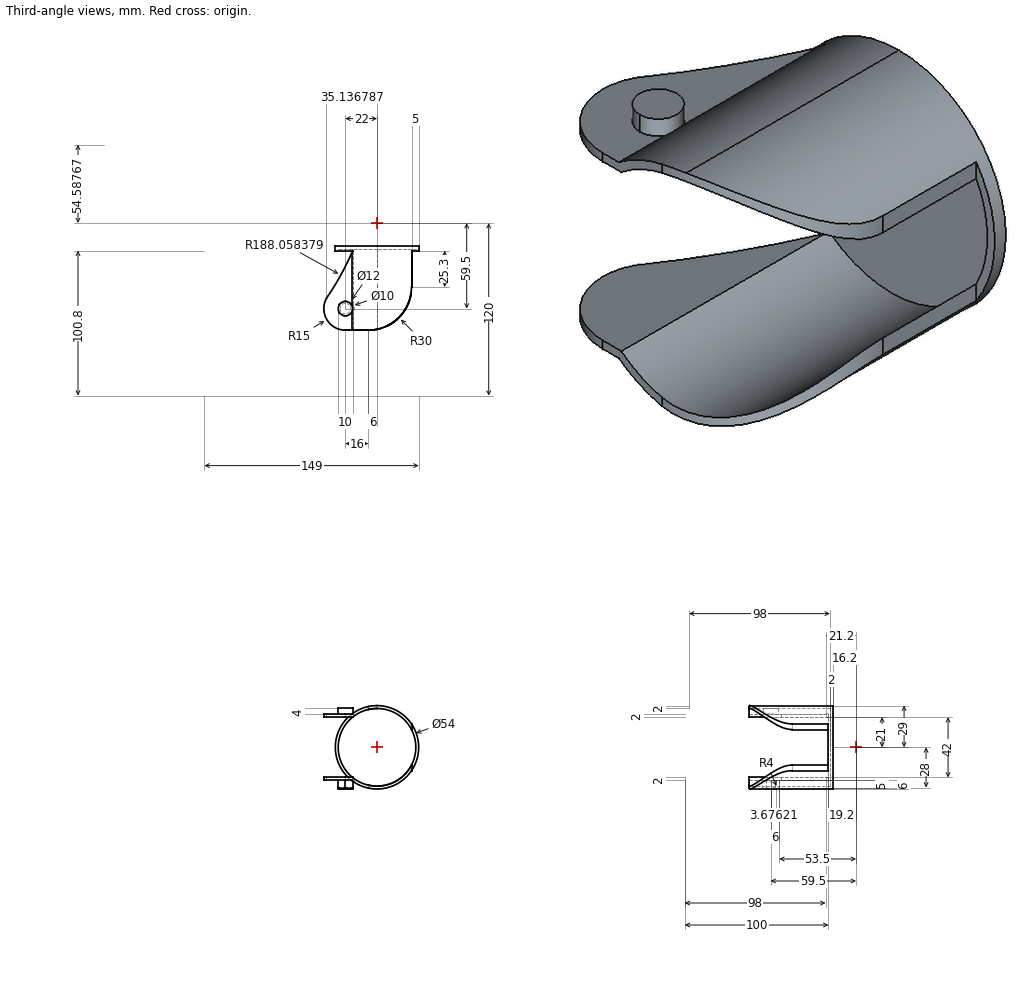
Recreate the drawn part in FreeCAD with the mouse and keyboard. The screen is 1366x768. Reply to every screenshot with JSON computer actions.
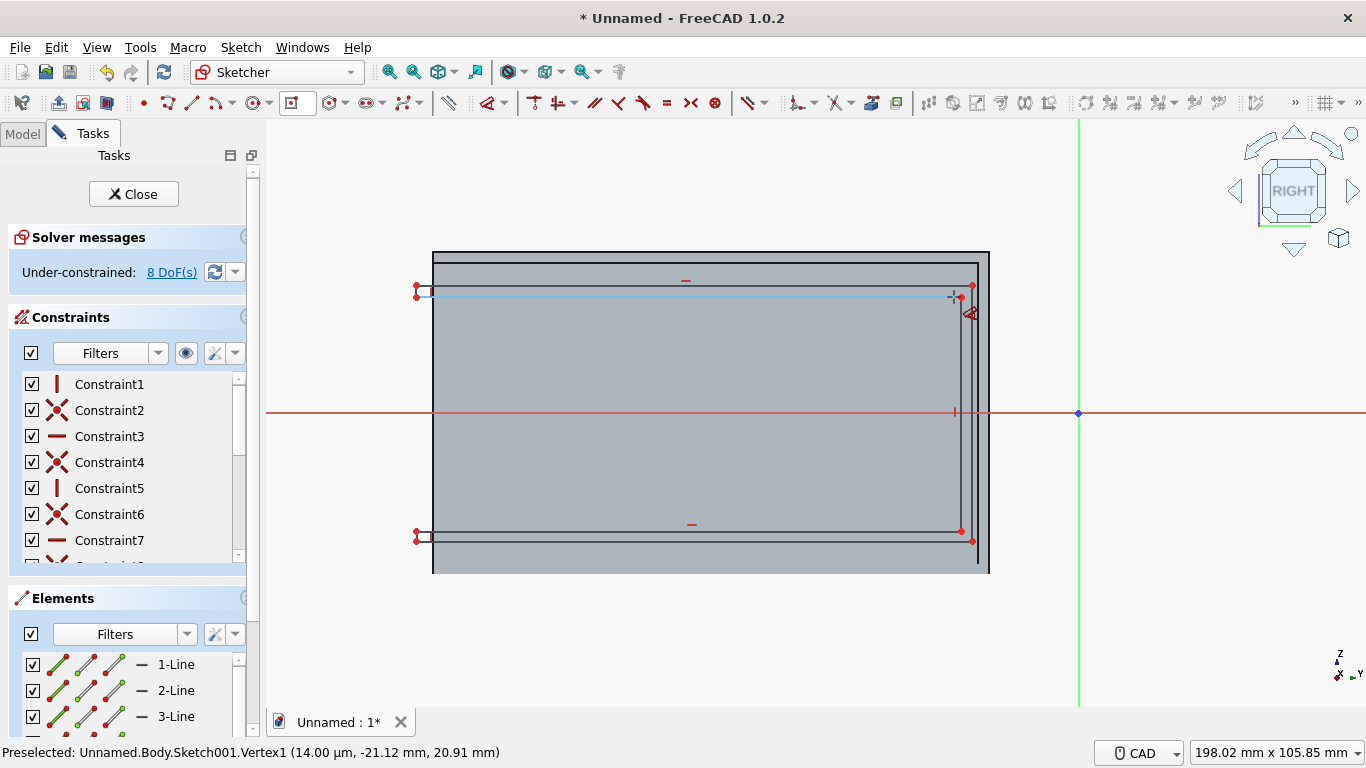
{"action": "scroll", "coordinate": [417, 537], "scroll_direction": "up", "scroll_amount": 7}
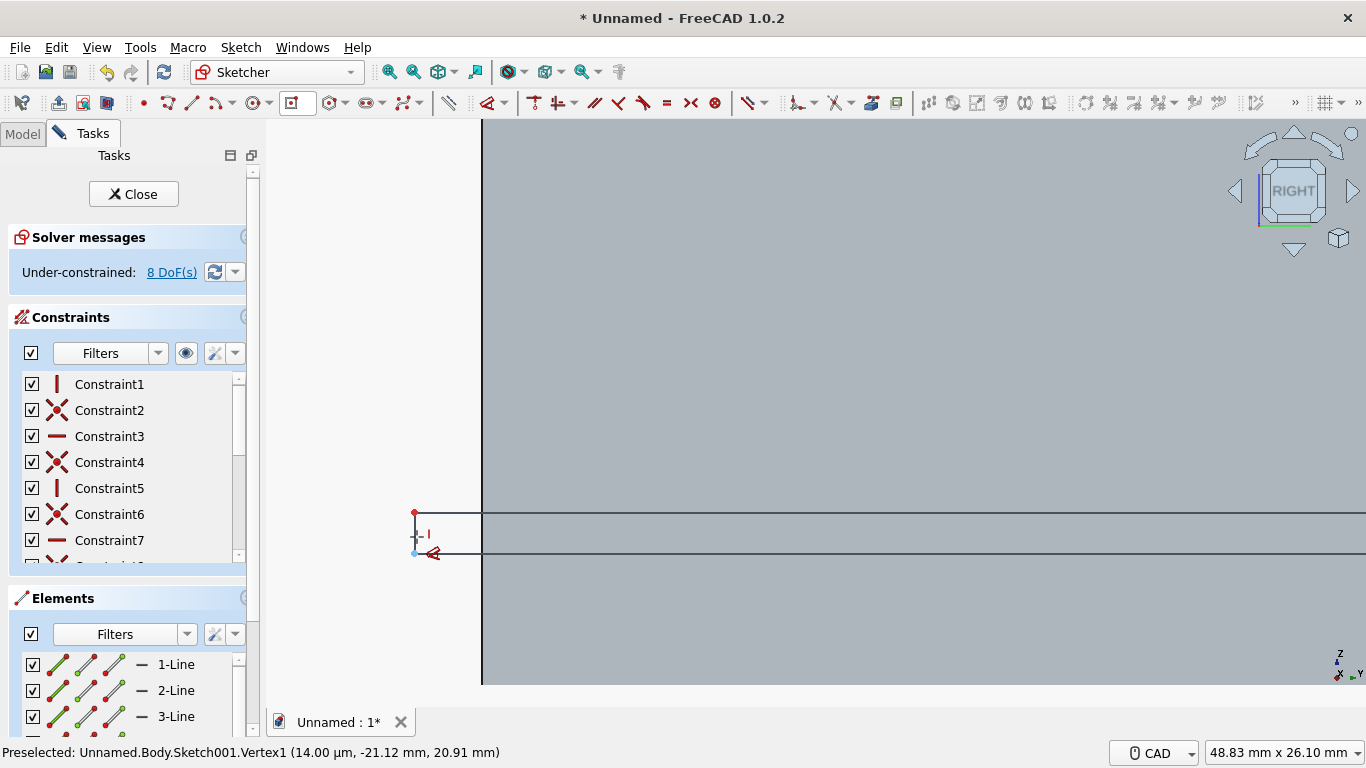
{"action": "left_click", "coordinate": [415, 533]}
{"action": "left_click", "coordinate": [381, 533]}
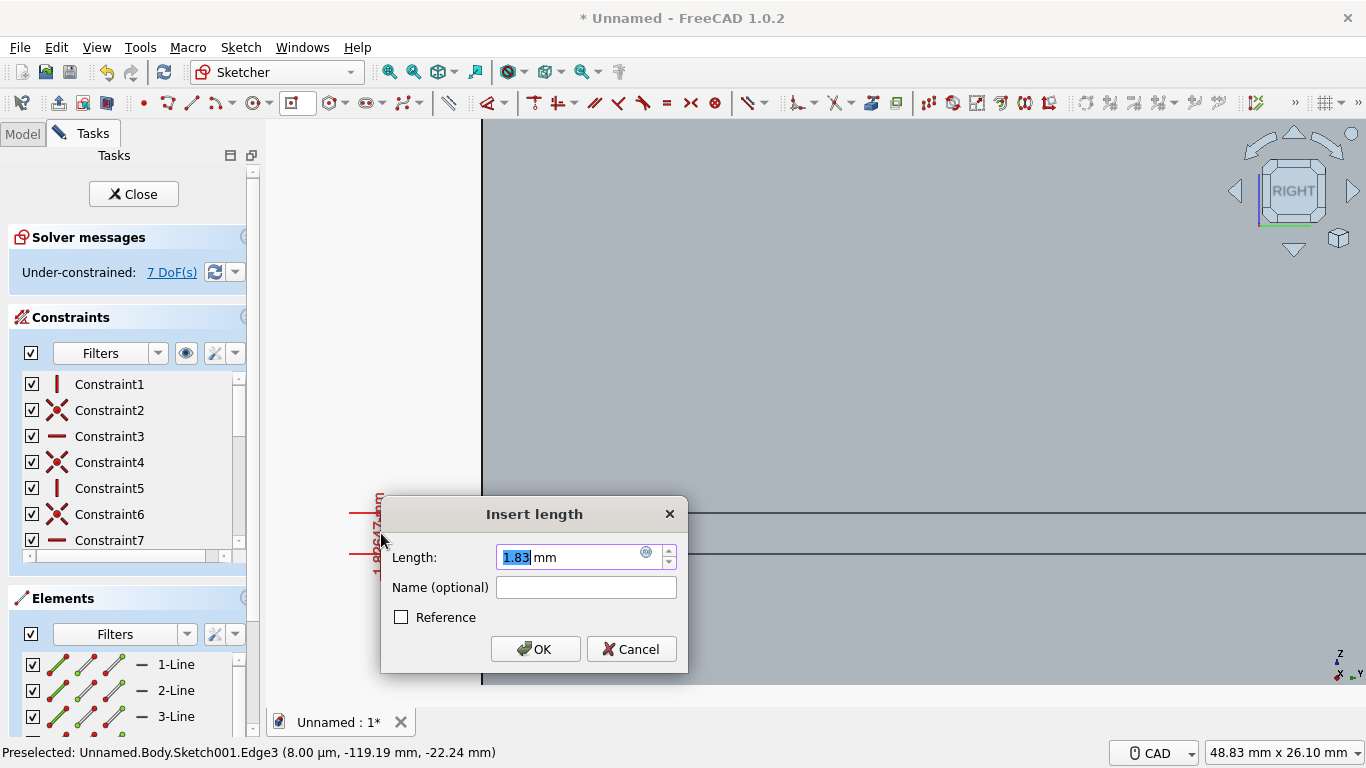
{"action": "type", "text": "2"}
{"action": "key", "text": "Return"}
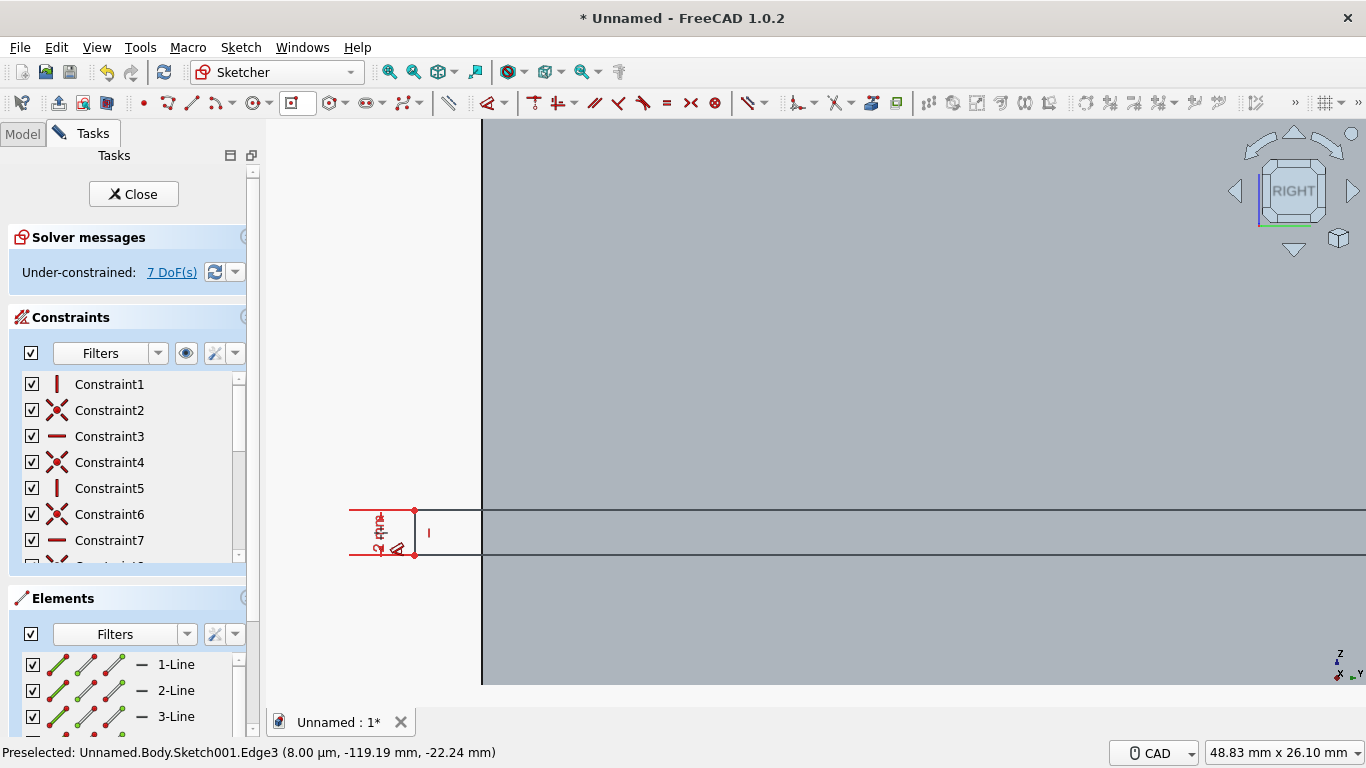
{"action": "scroll", "coordinate": [417, 537], "scroll_direction": "down", "scroll_amount": 7}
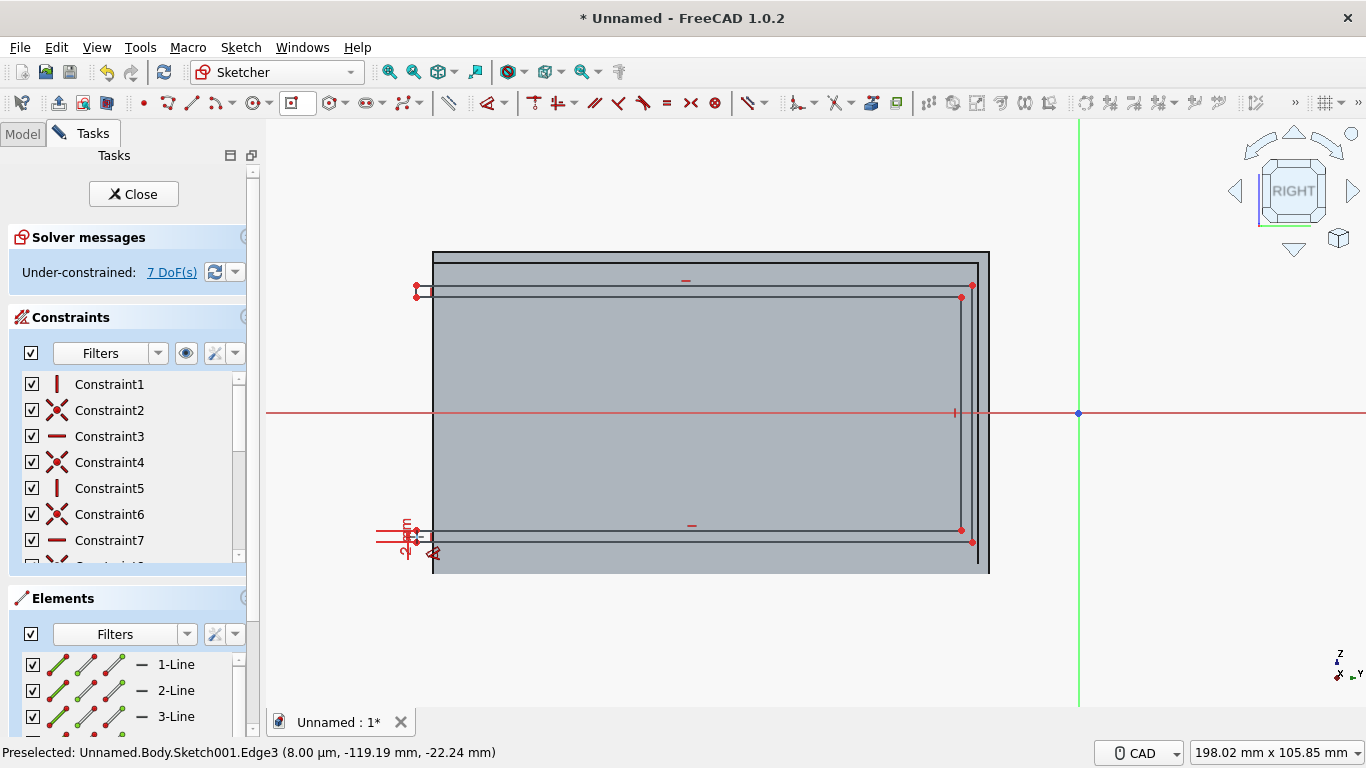
{"action": "scroll", "coordinate": [416, 289], "scroll_direction": "up", "scroll_amount": 8}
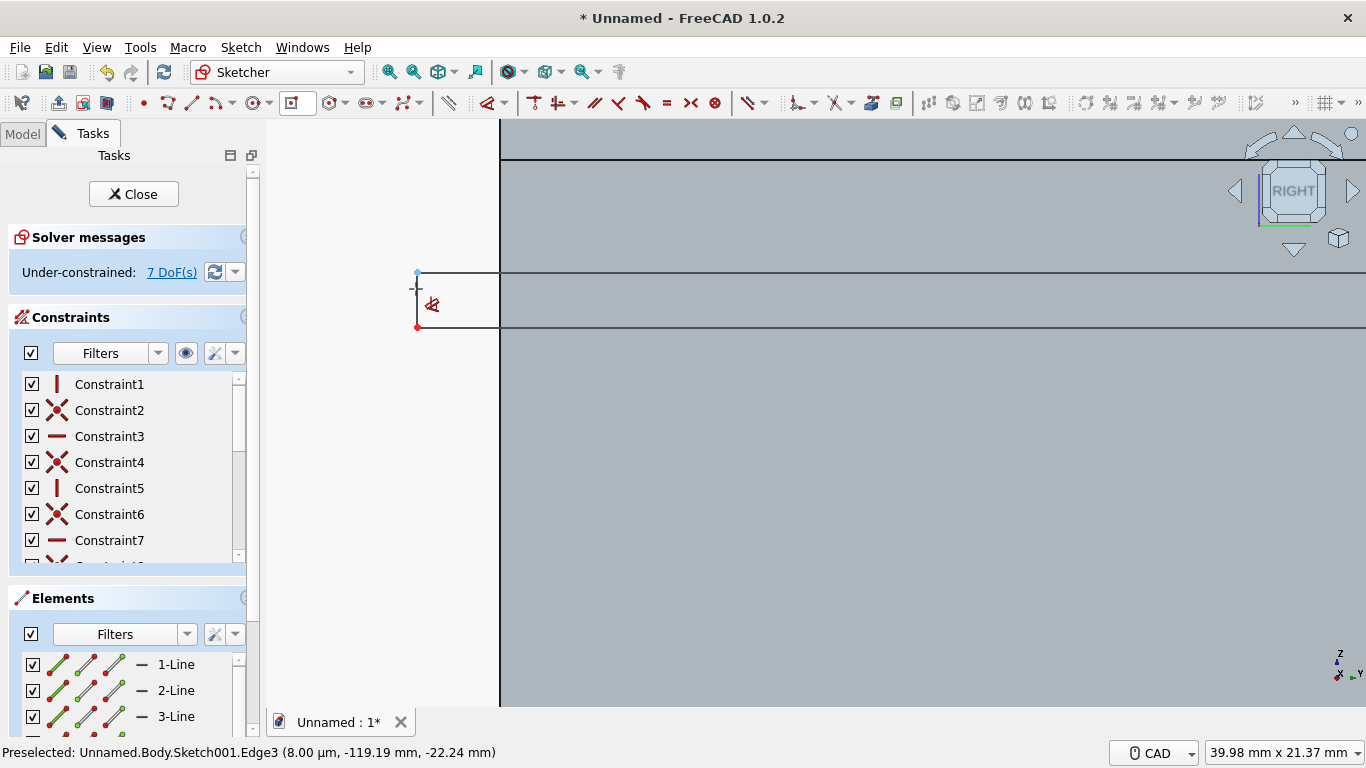
{"action": "left_click", "coordinate": [417, 289]}
{"action": "left_click", "coordinate": [383, 300]}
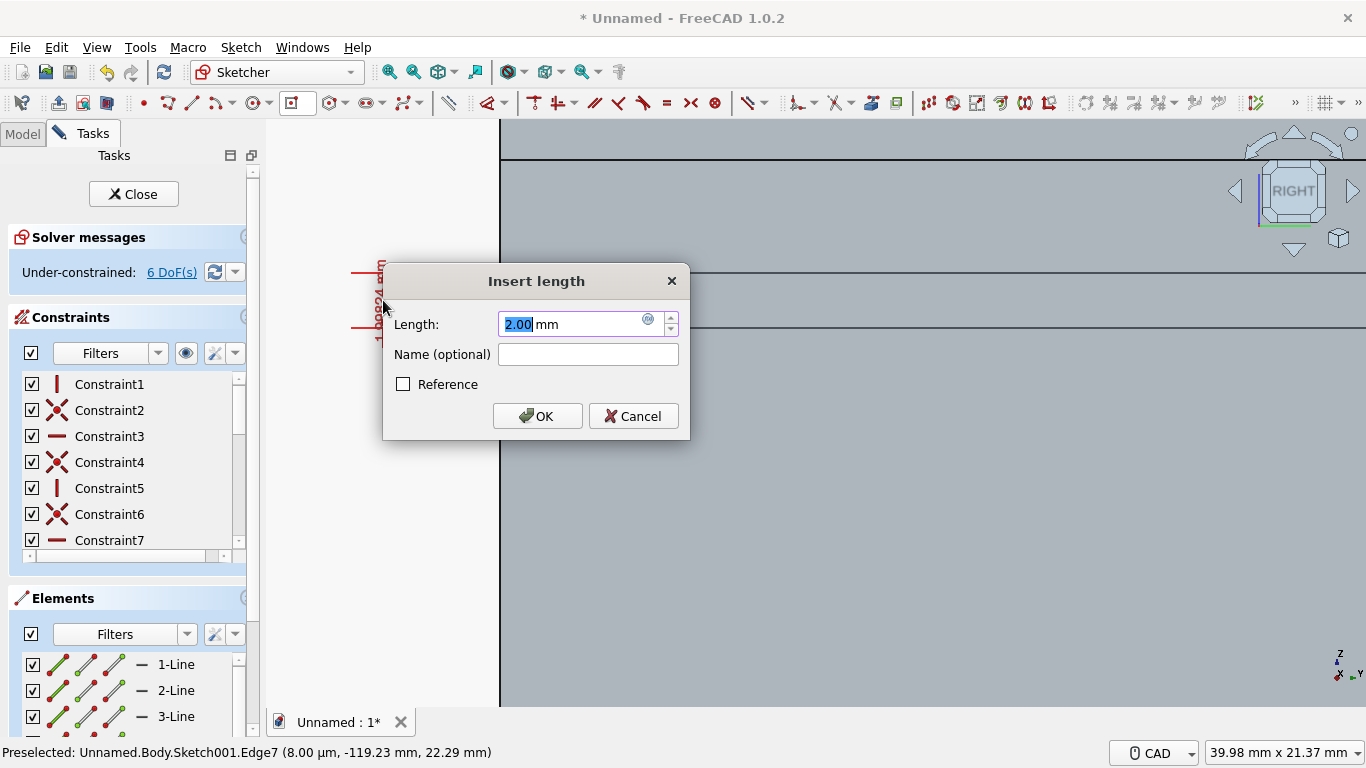
{"action": "type", "text": "2"}
{"action": "key", "text": "Return"}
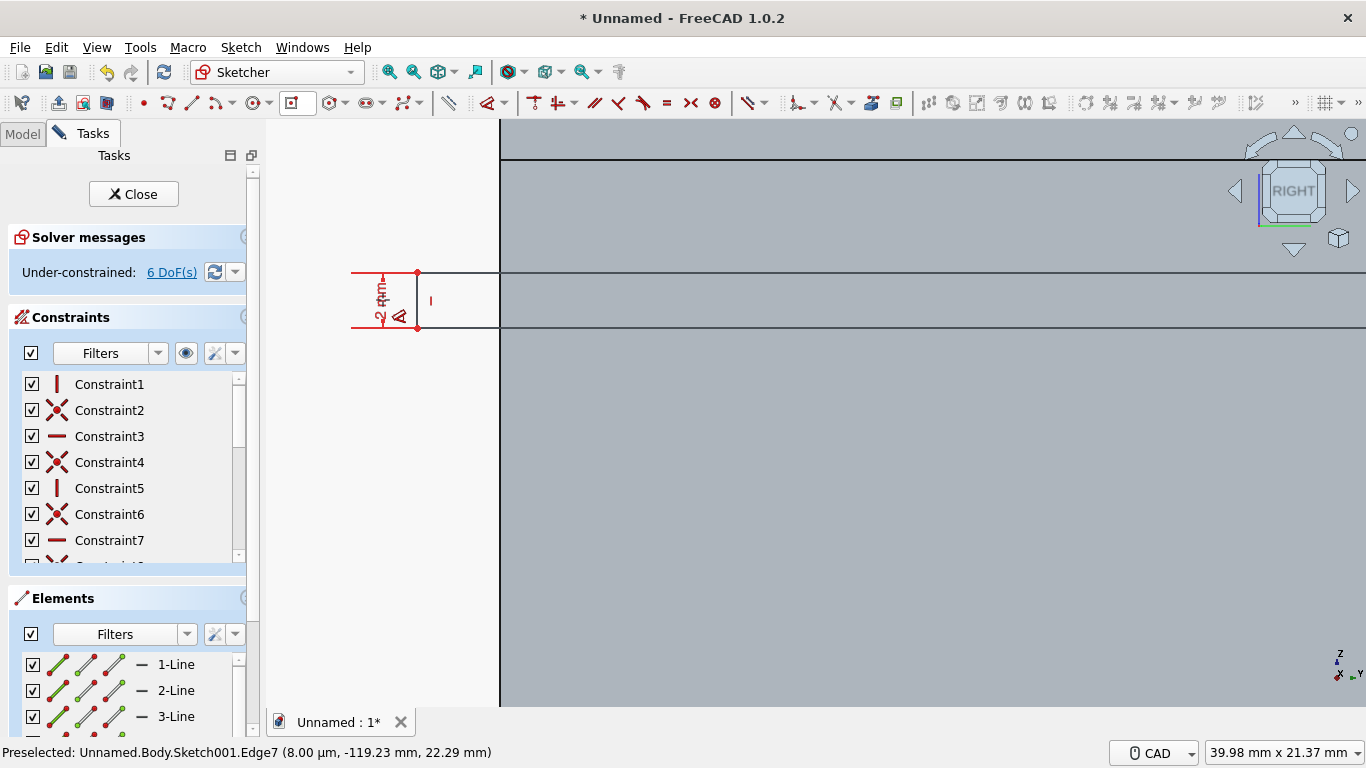
{"action": "scroll", "coordinate": [416, 289], "scroll_direction": "down", "scroll_amount": 8}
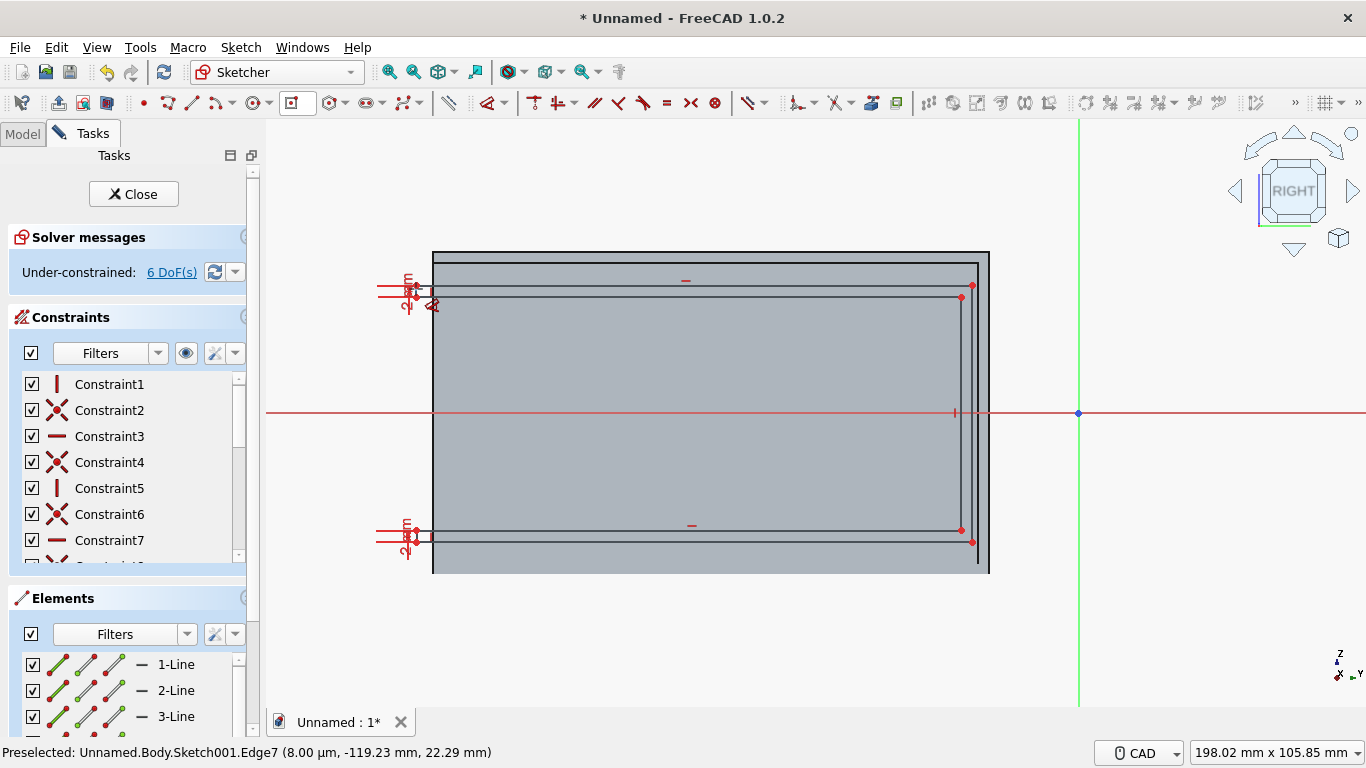
{"action": "scroll", "coordinate": [961, 367], "scroll_direction": "up", "scroll_amount": 2}